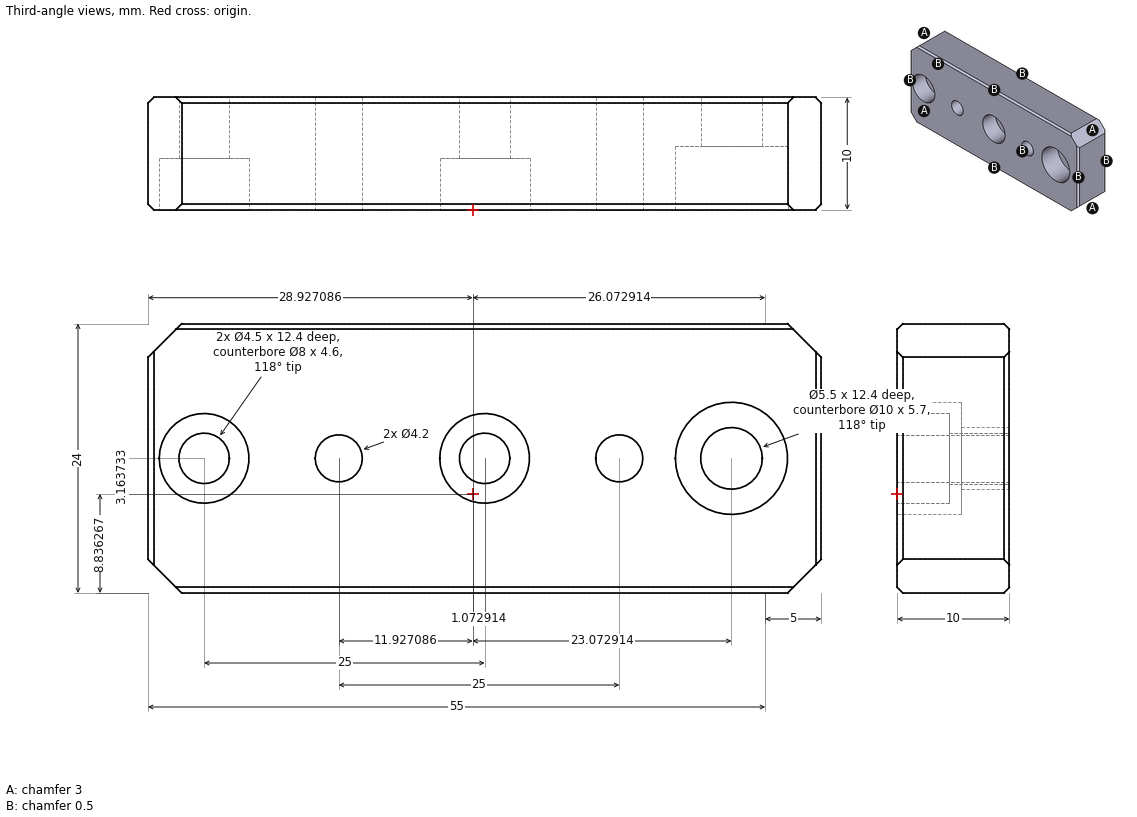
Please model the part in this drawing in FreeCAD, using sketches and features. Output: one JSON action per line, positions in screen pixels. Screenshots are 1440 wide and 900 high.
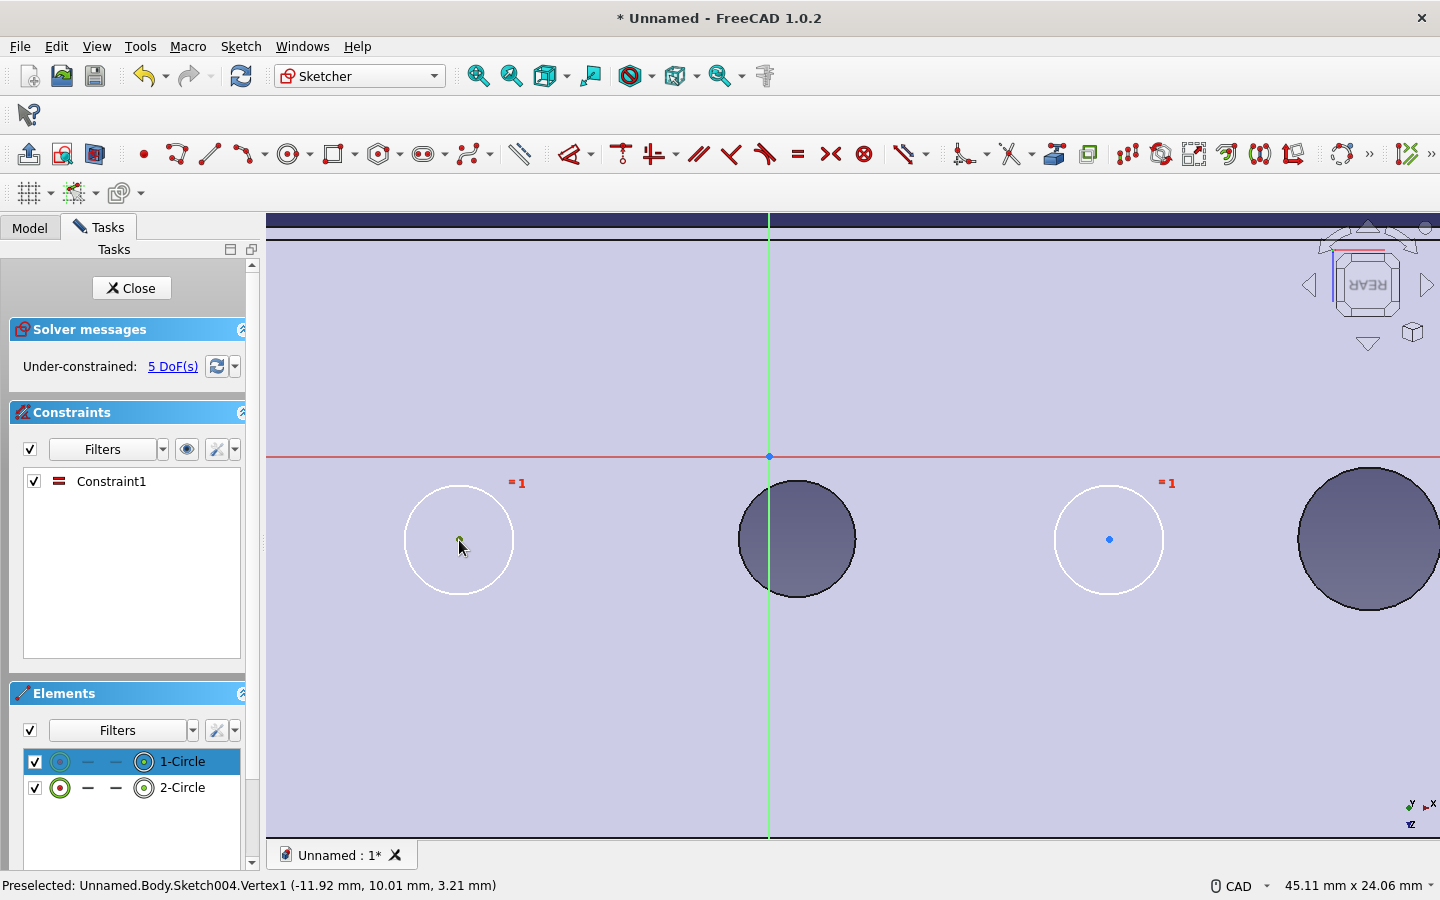
{"action": "left_click", "coordinate": [1109, 540]}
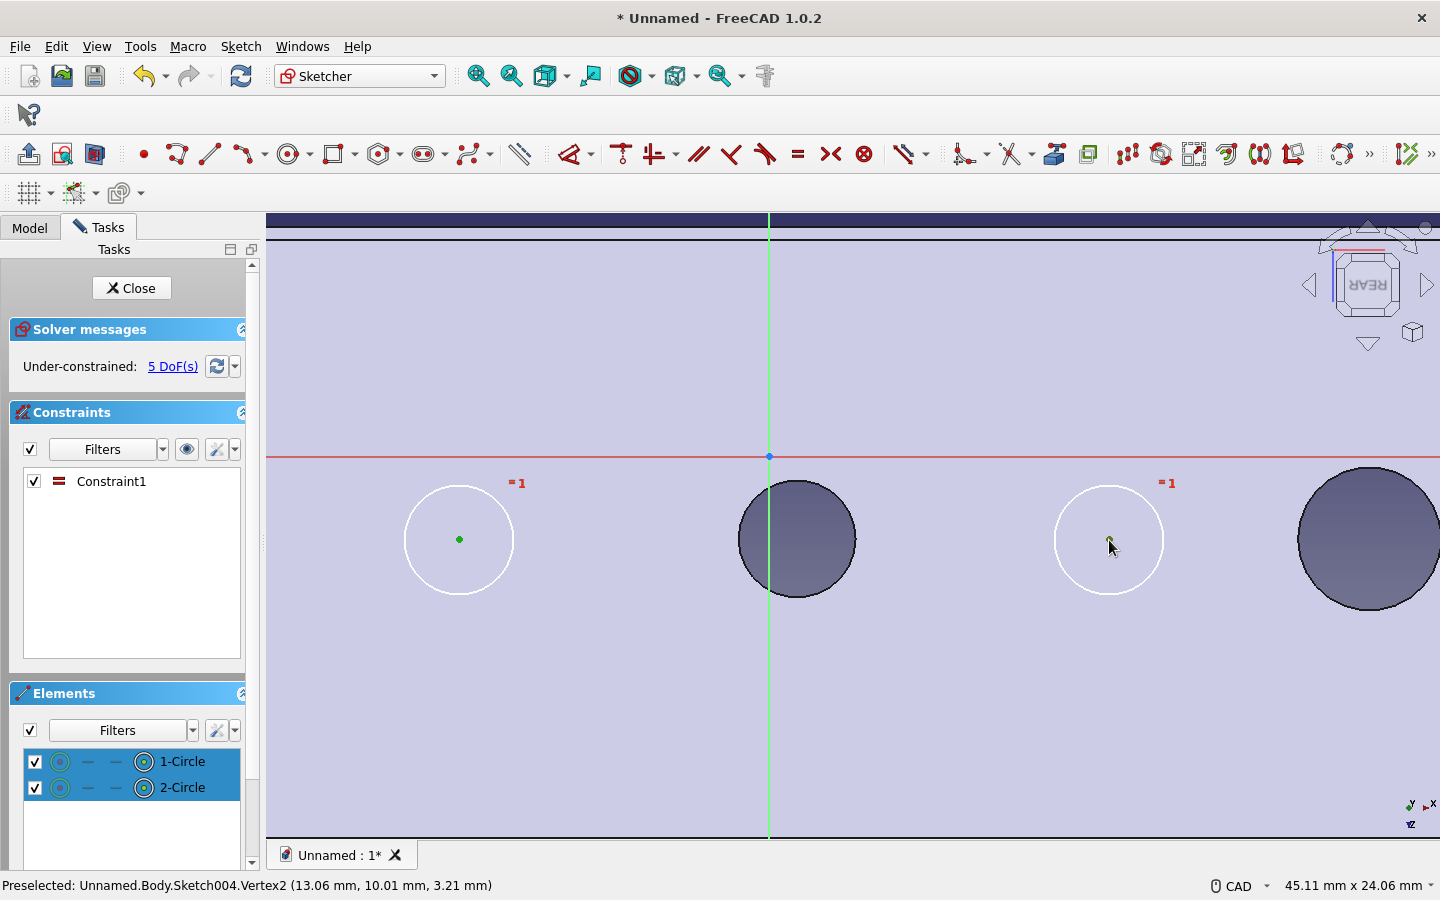
{"action": "key", "text": "h"}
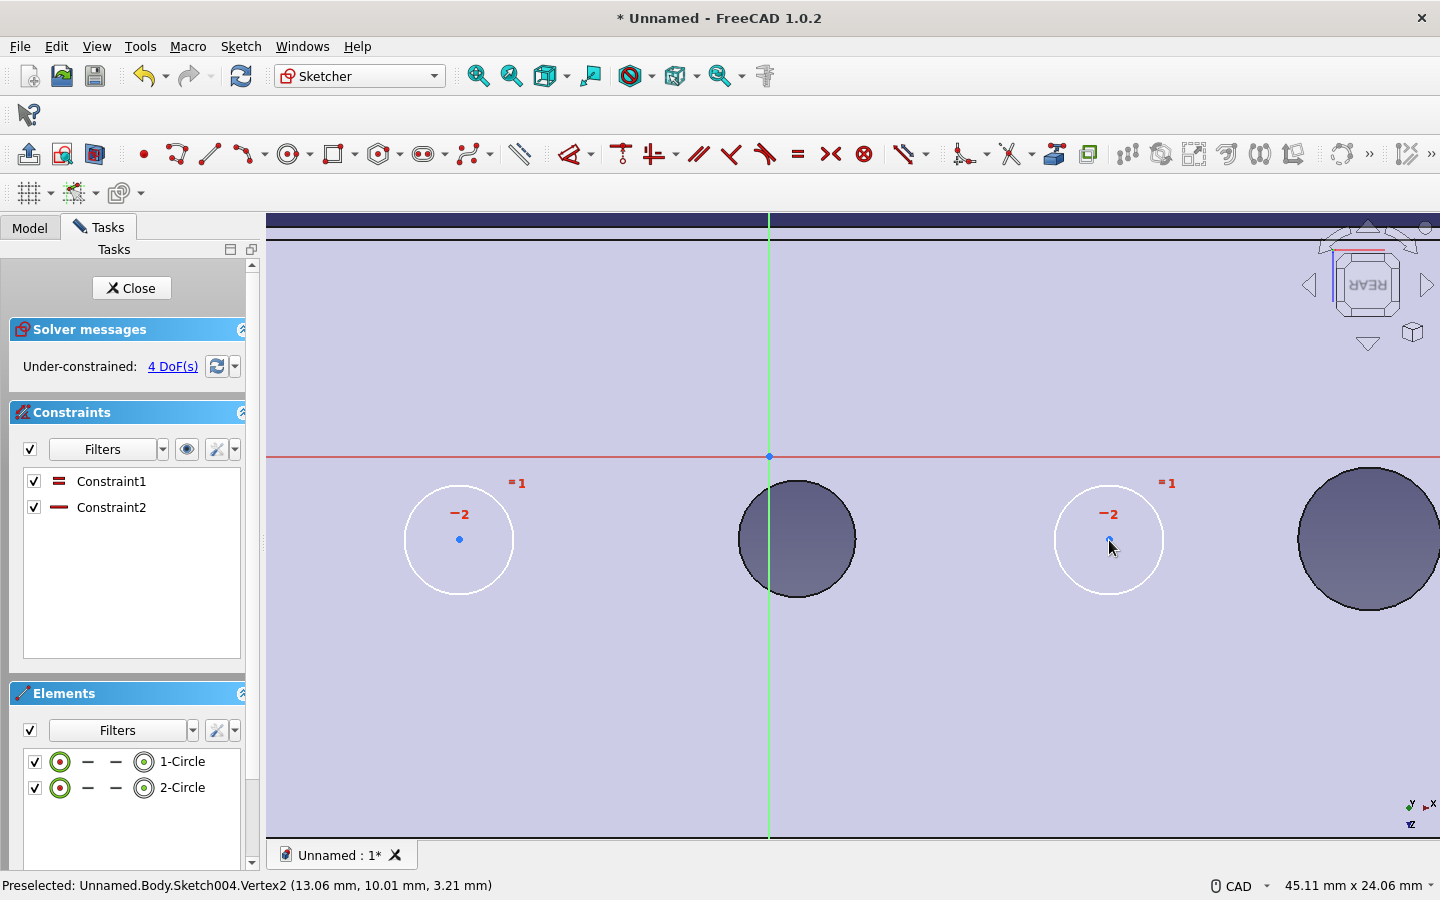
{"action": "key", "text": "d"}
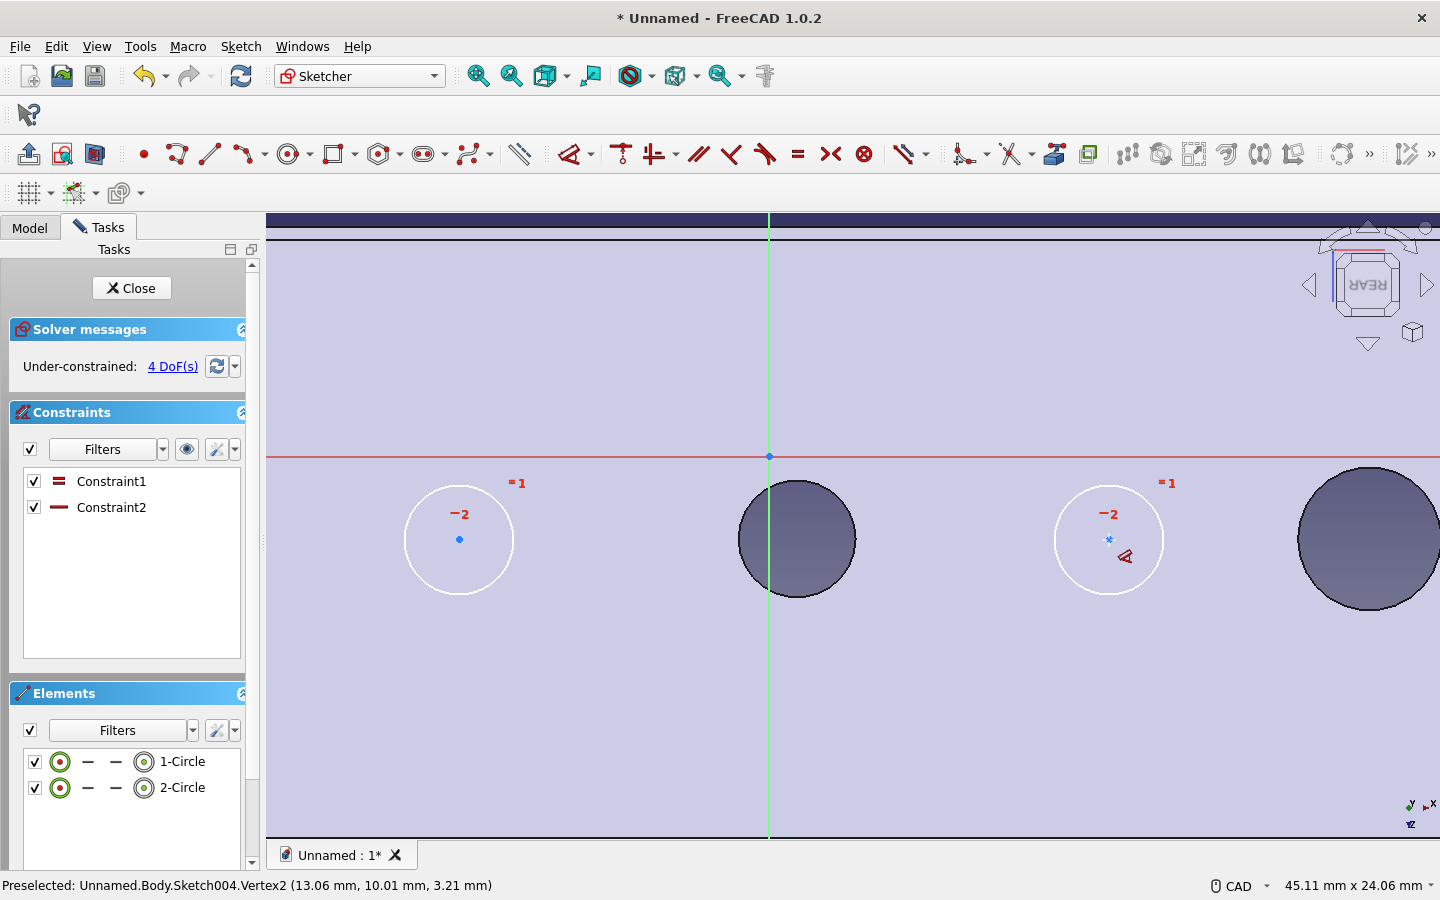
{"action": "left_click", "coordinate": [497, 501]}
{"action": "left_click", "coordinate": [519, 478]}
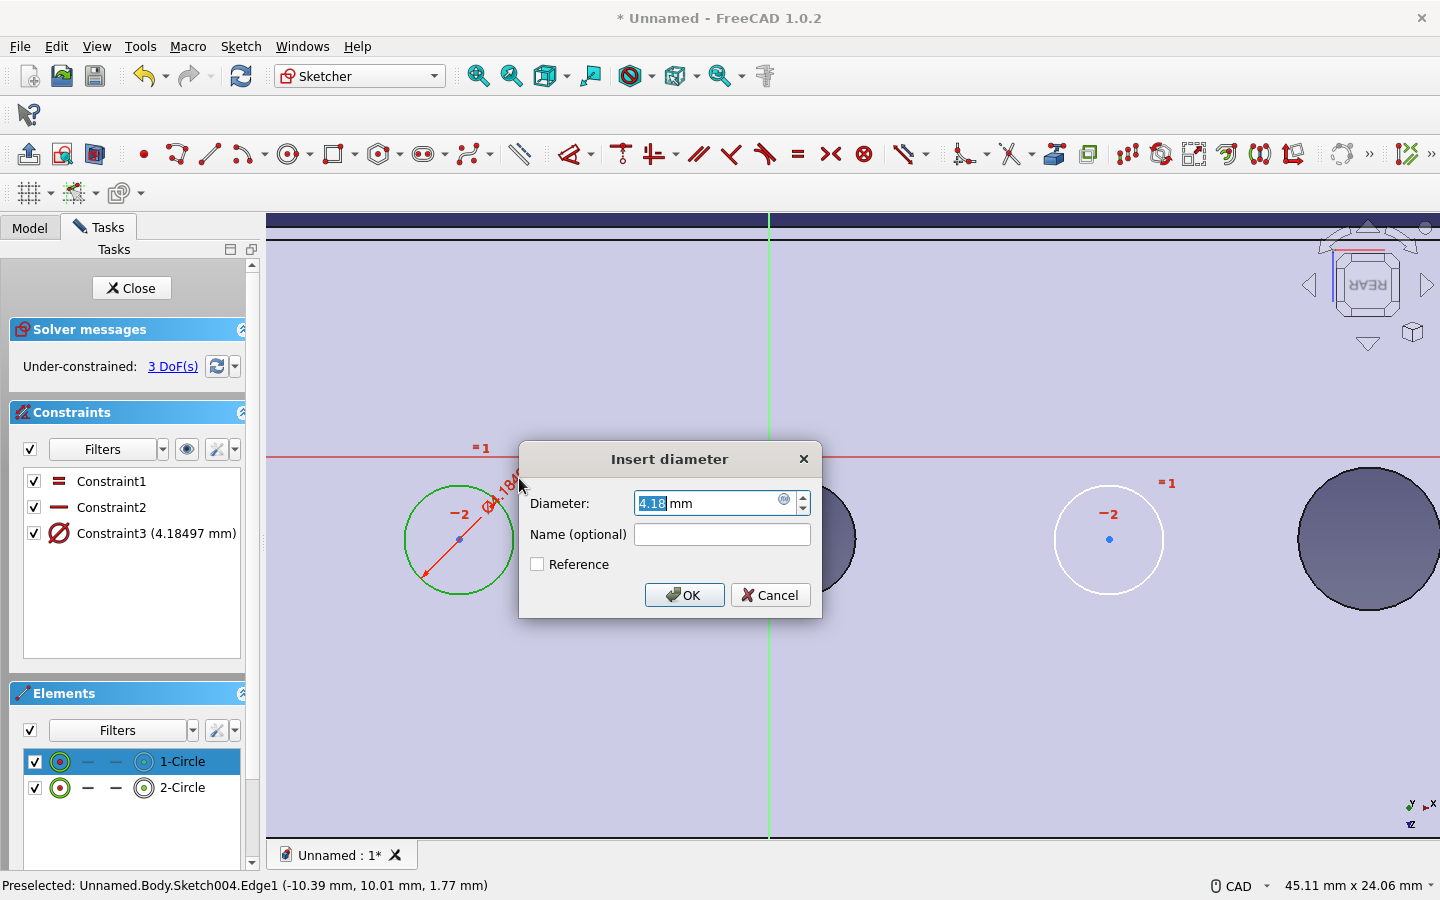
{"action": "type", "text": "4.2"}
{"action": "key", "text": "Return"}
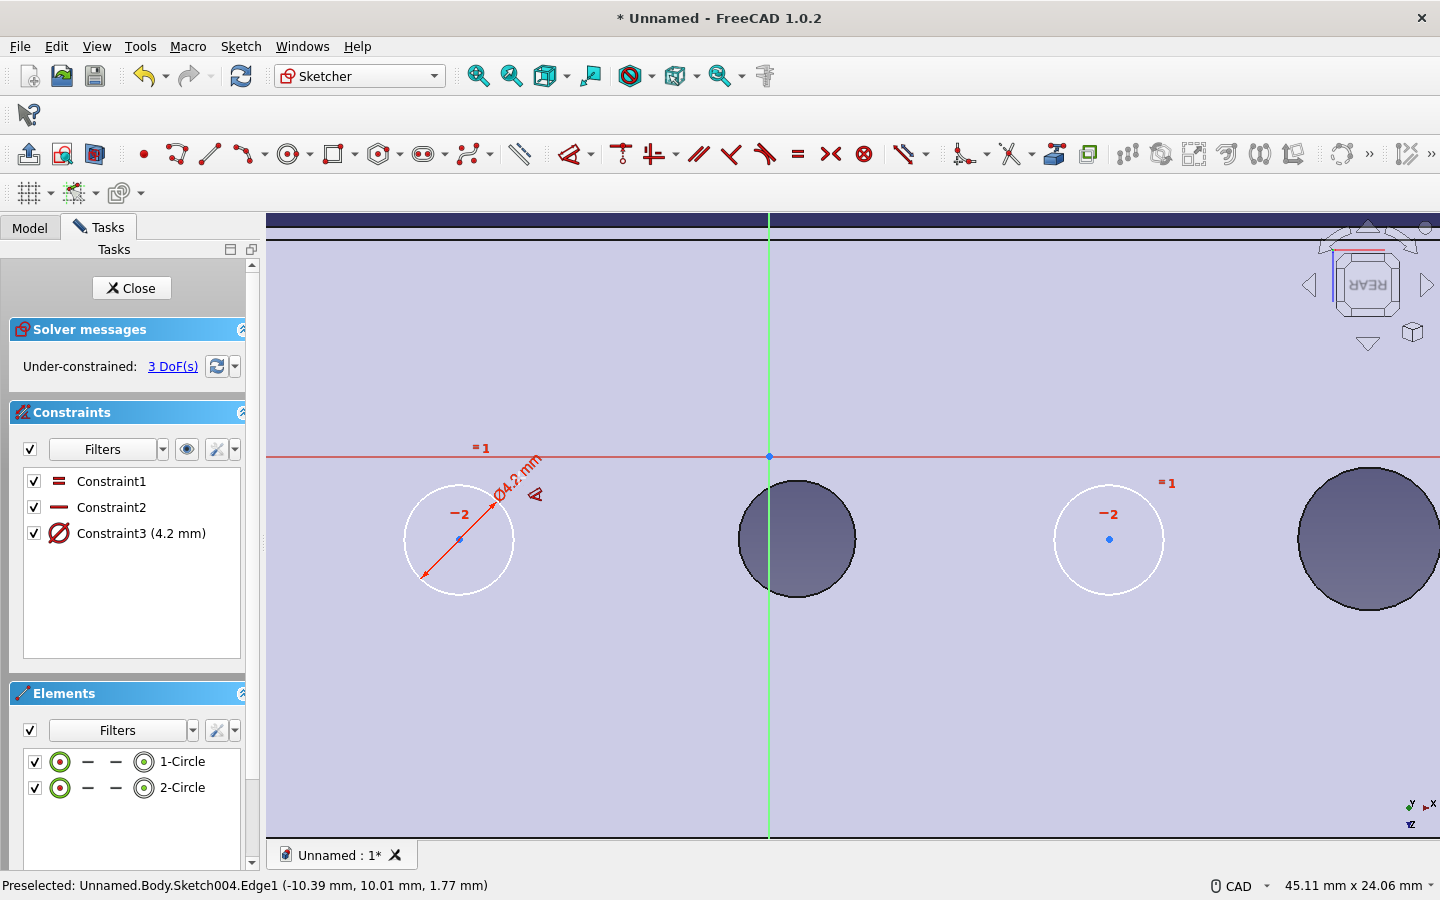
{"action": "left_click", "coordinate": [459, 540]}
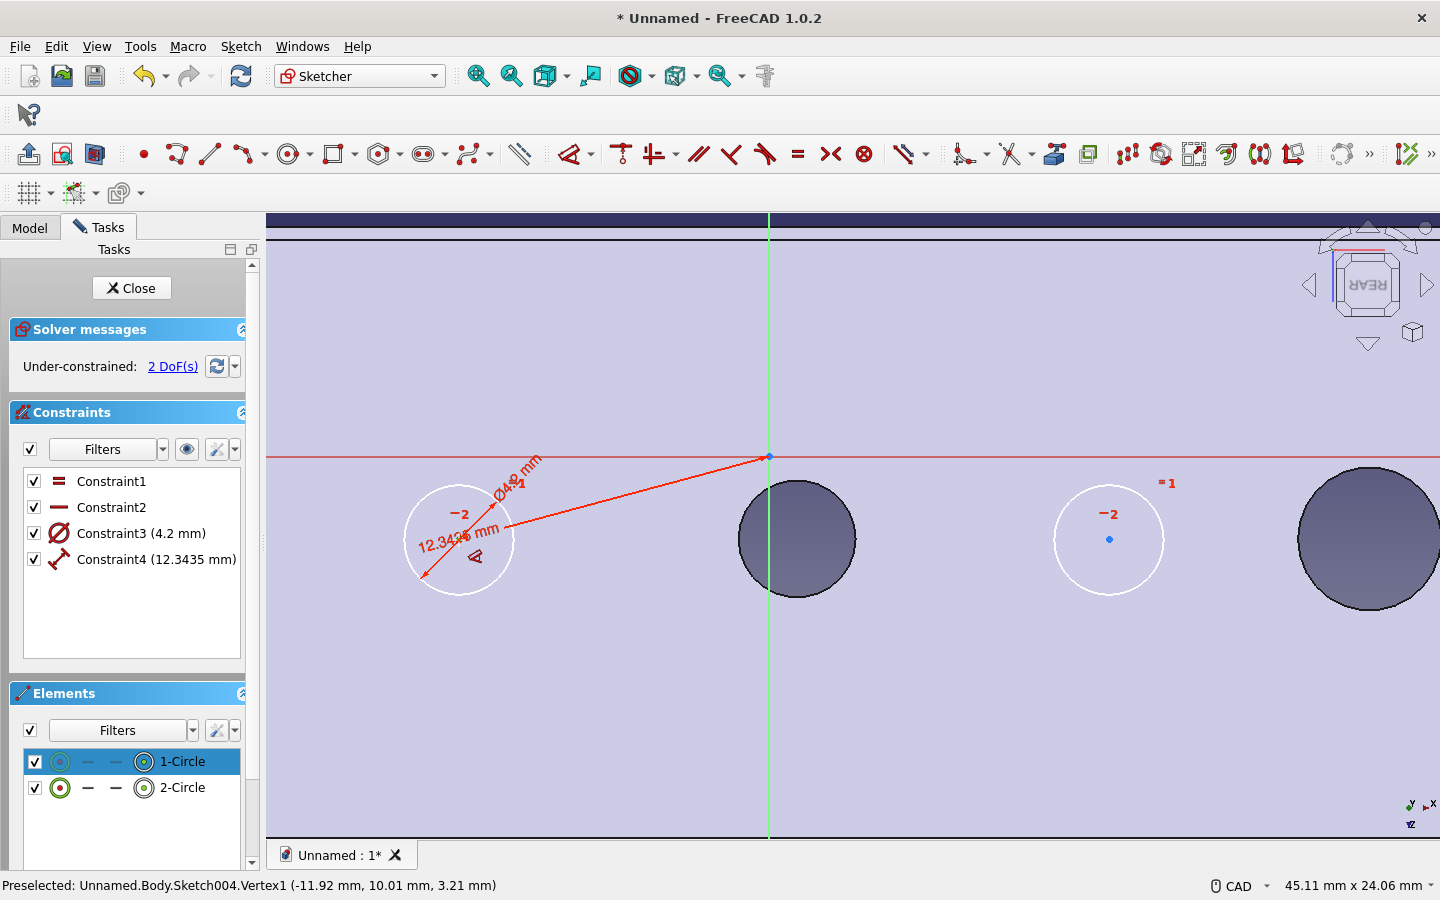
{"action": "left_click", "coordinate": [1109, 540]}
{"action": "left_click", "coordinate": [784, 574]}